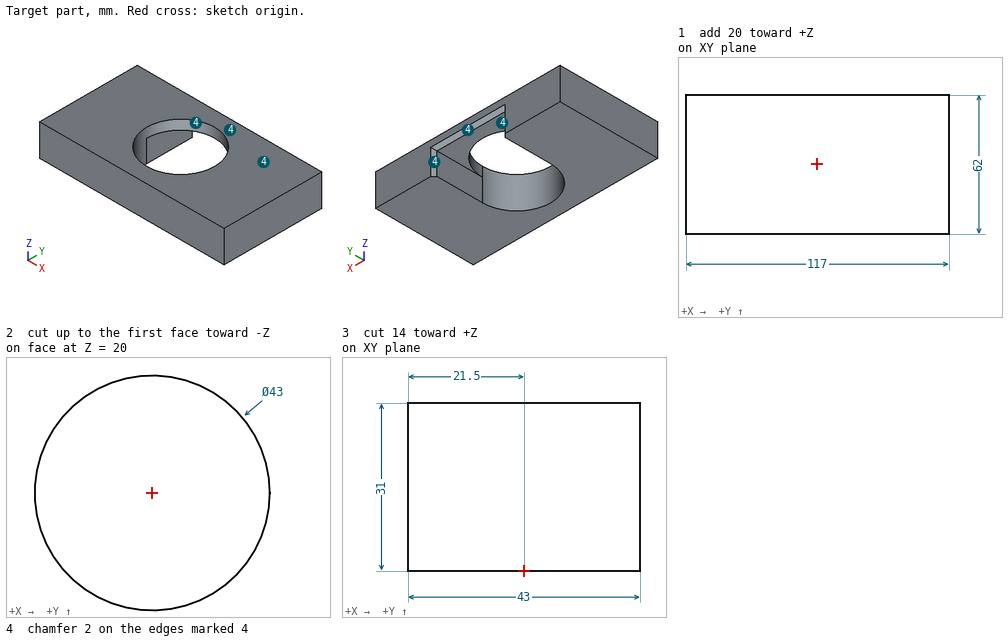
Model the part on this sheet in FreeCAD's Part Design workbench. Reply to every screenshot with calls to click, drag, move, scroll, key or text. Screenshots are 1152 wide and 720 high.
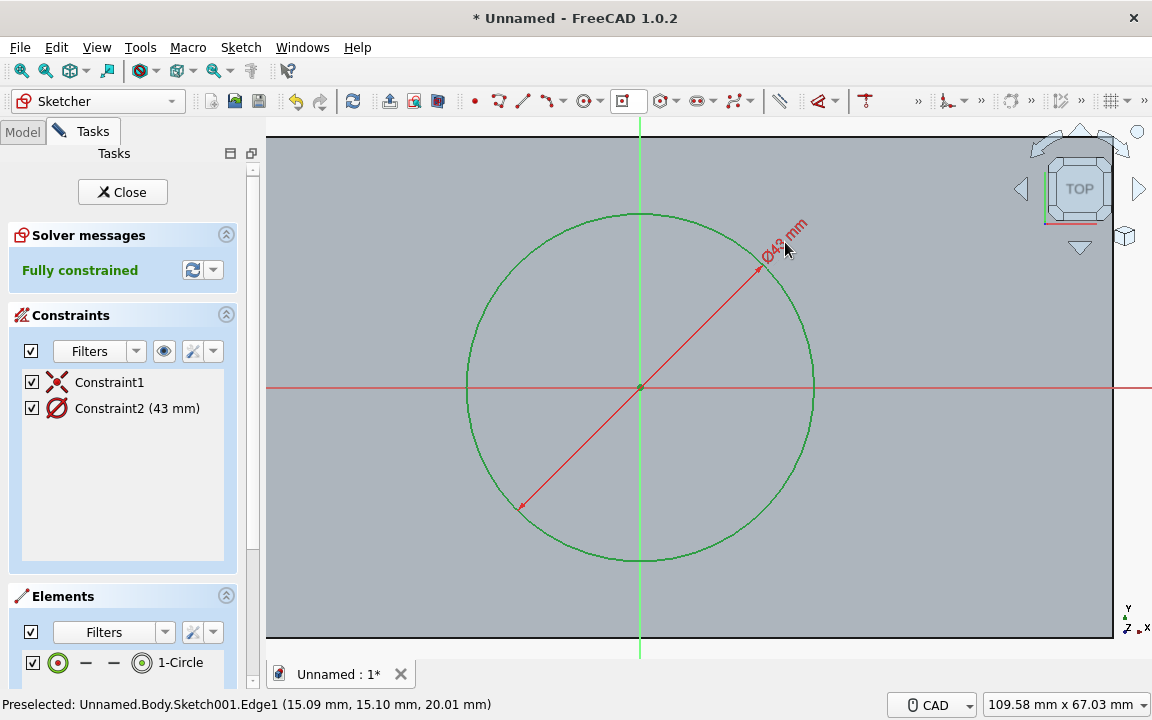
click(123, 192)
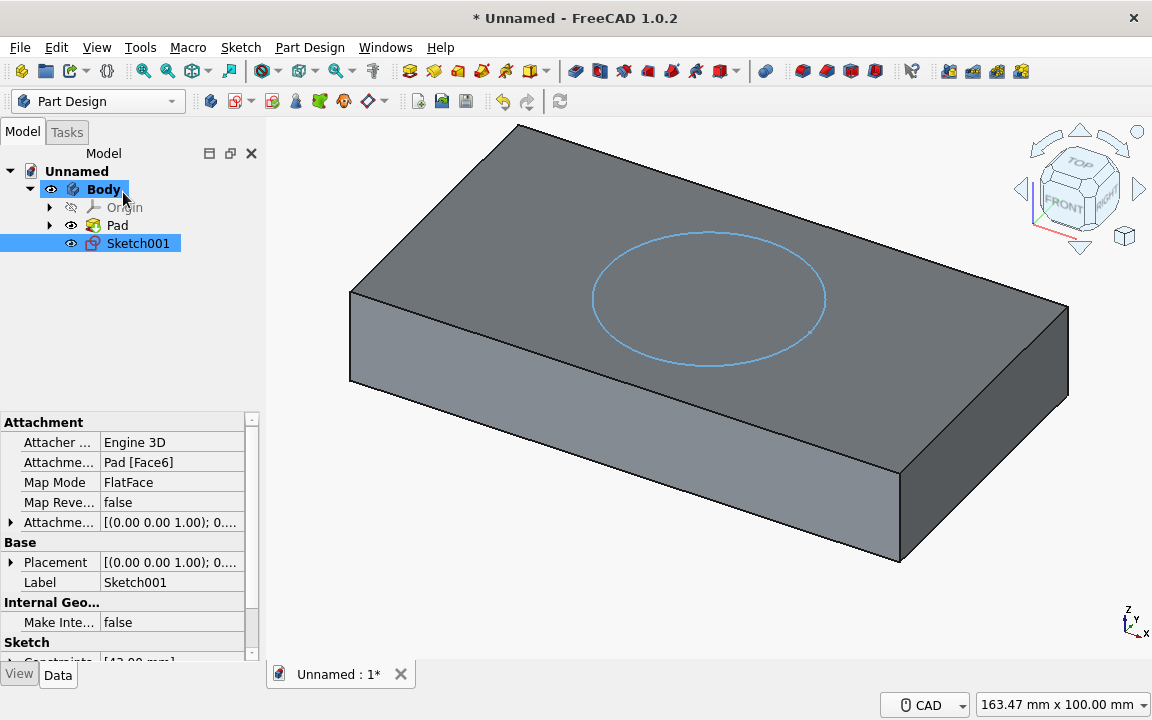
click(576, 72)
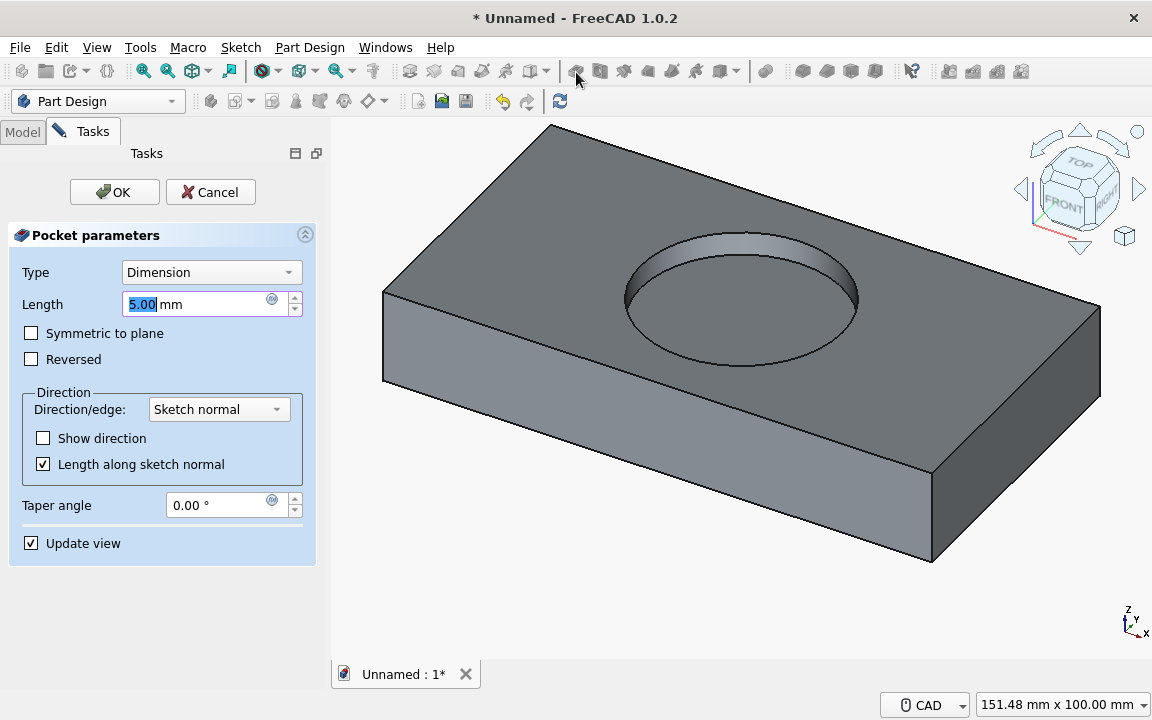
click(212, 272)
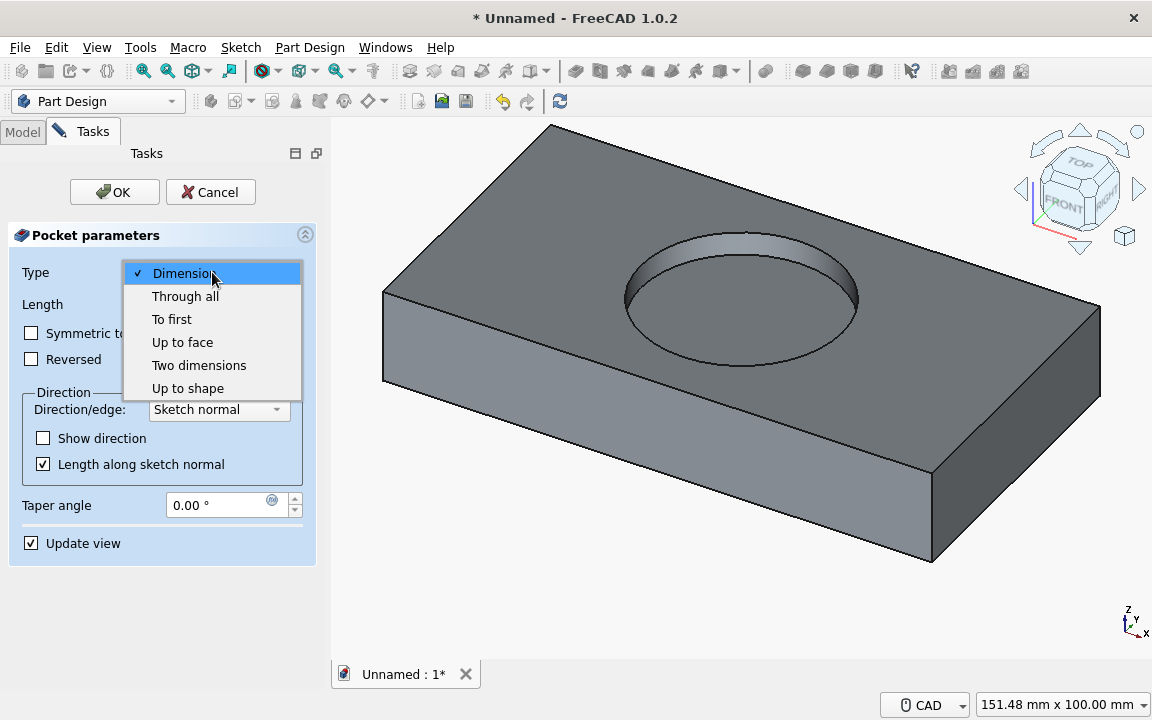
click(212, 320)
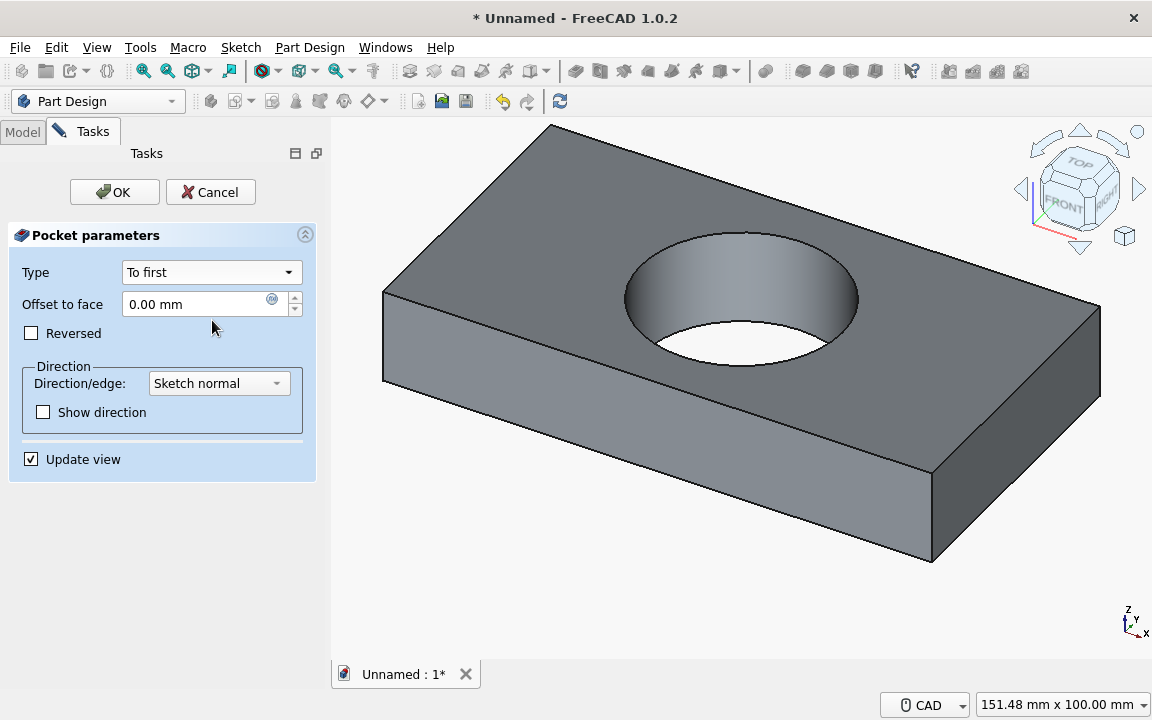
click(115, 192)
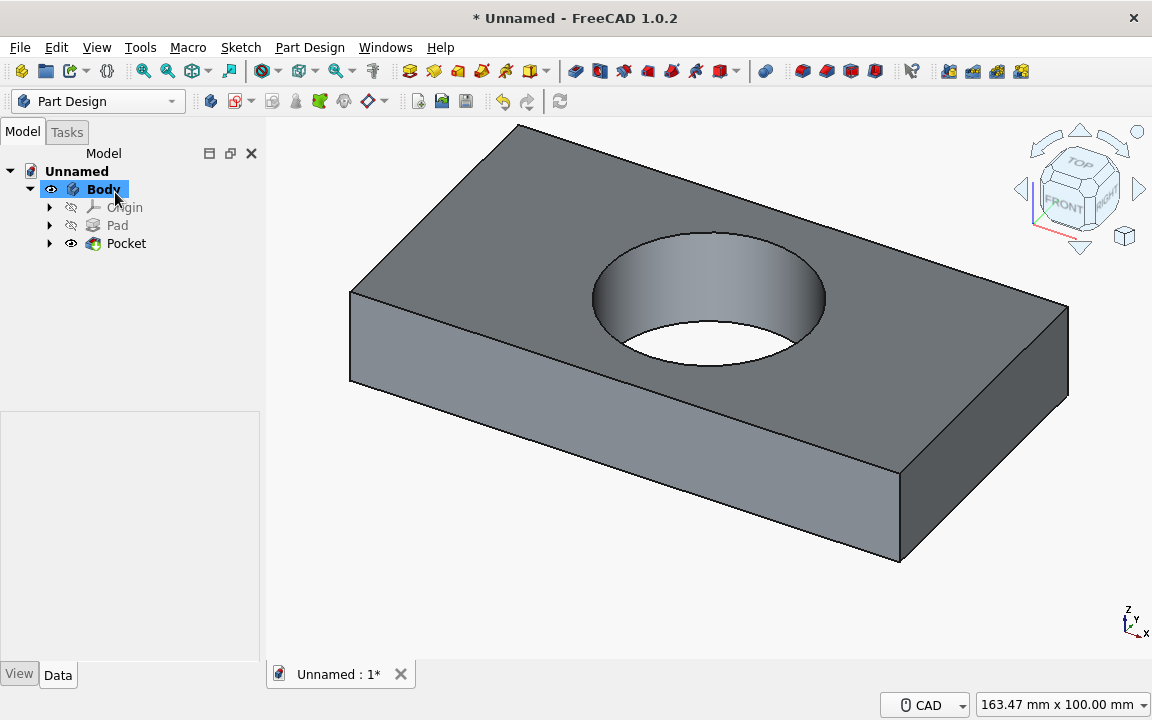
click(236, 102)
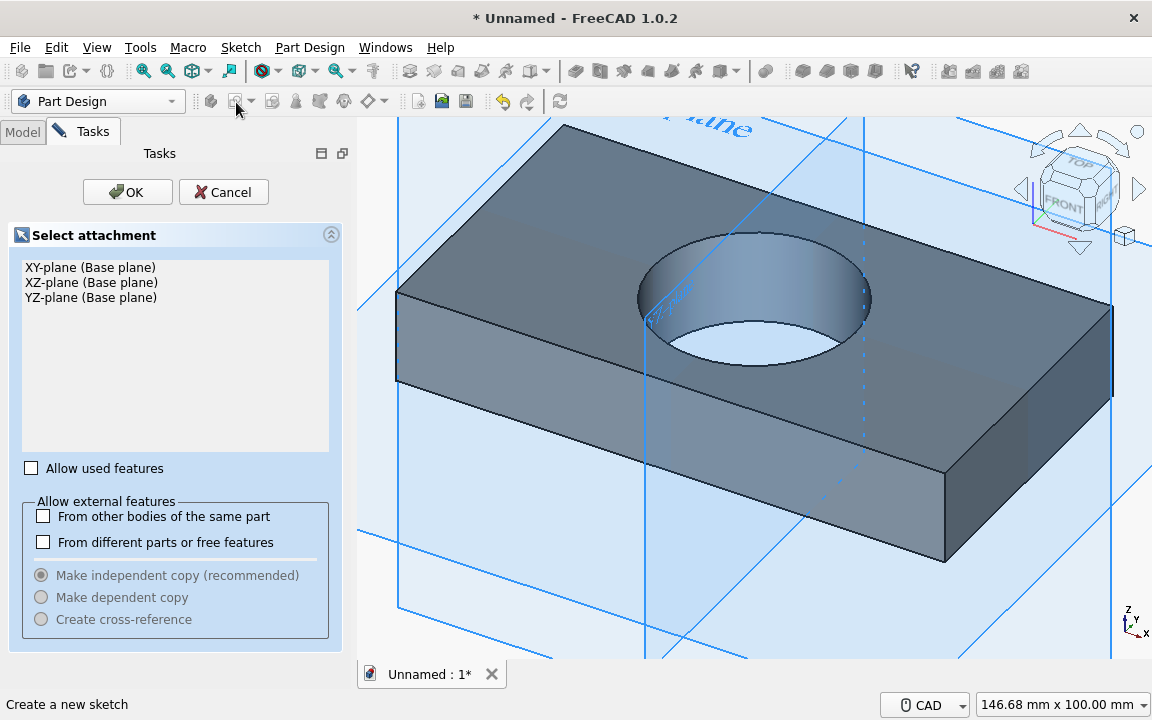
click(82, 268)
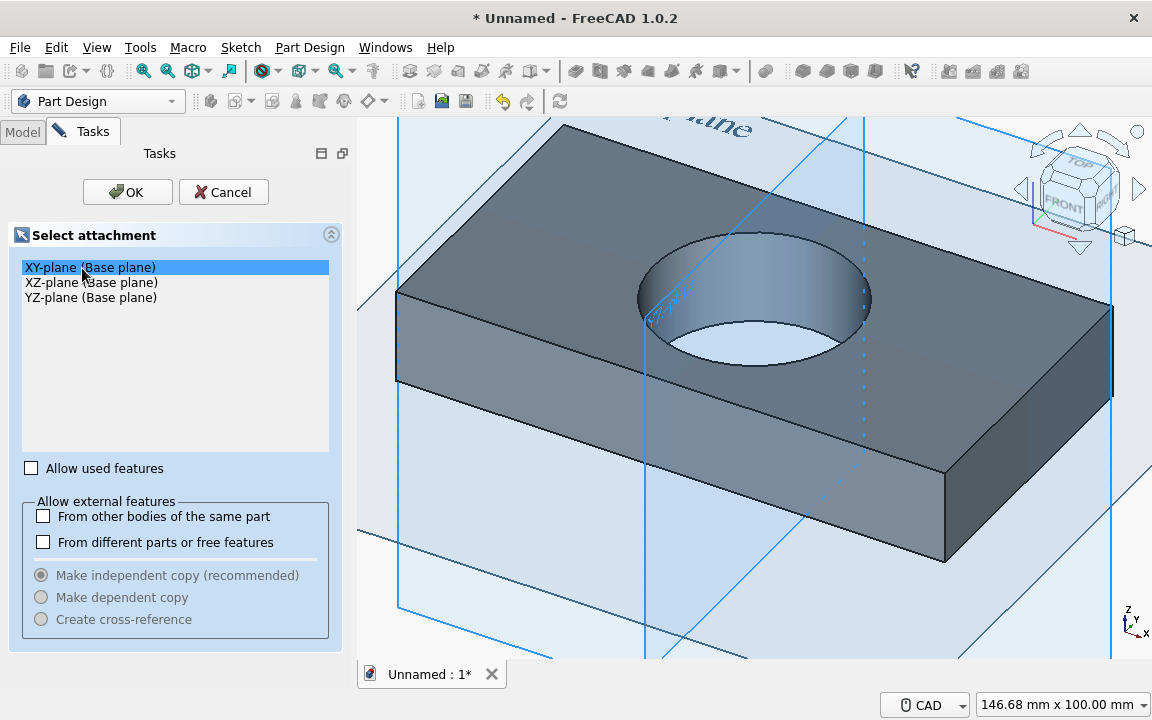
click(128, 192)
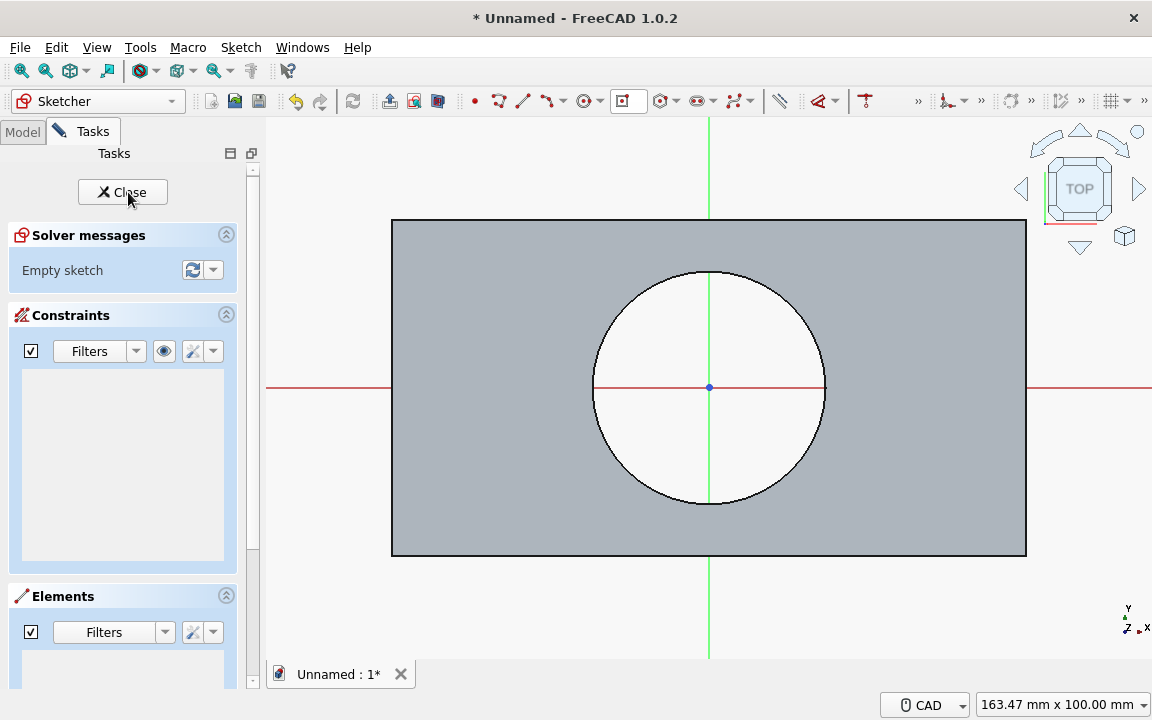
key(q)
key(s)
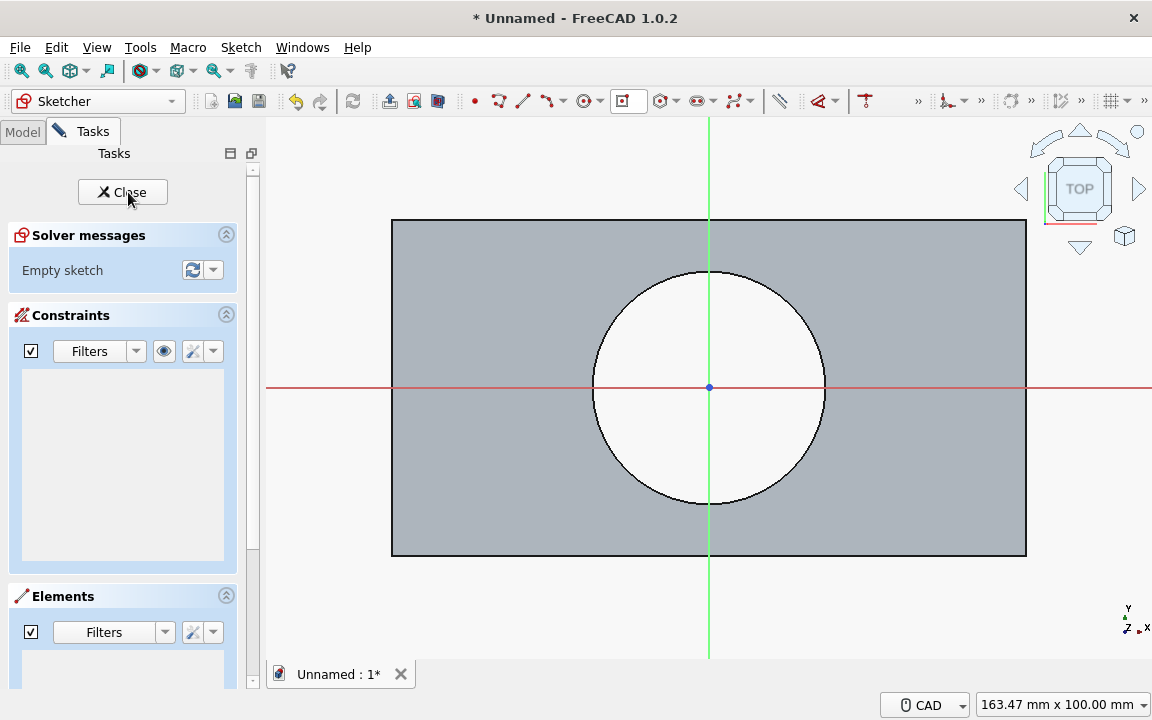
scroll(765, 235, up, 4)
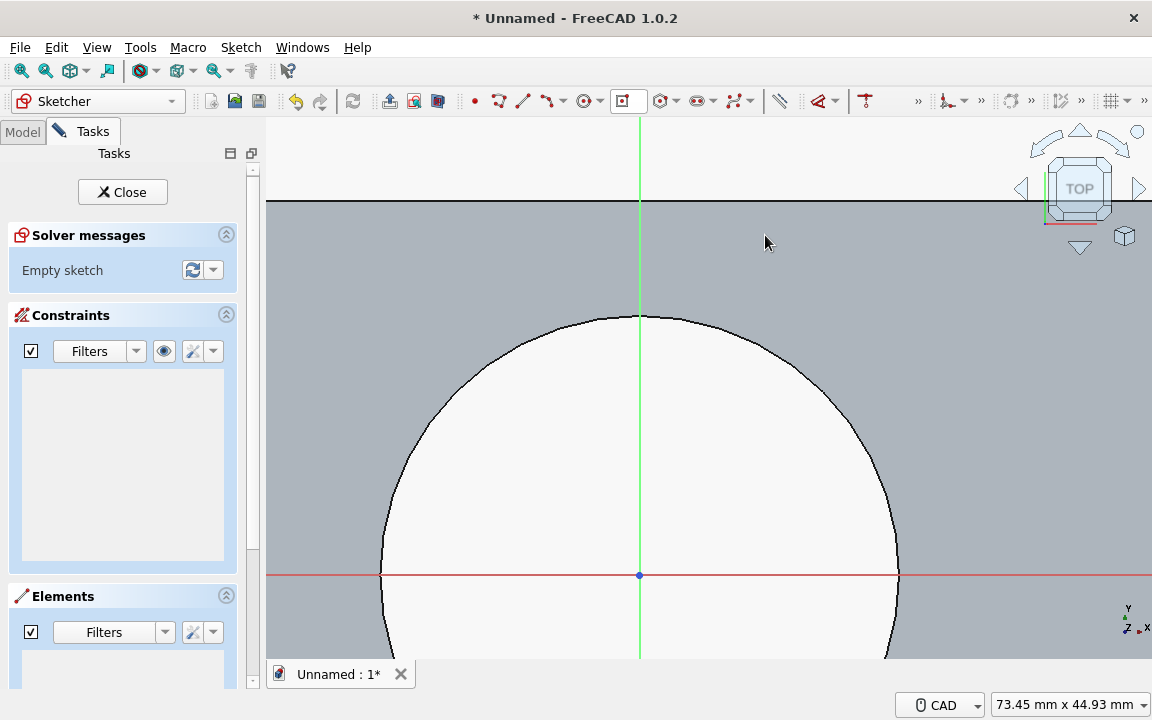
key(g)
key(r)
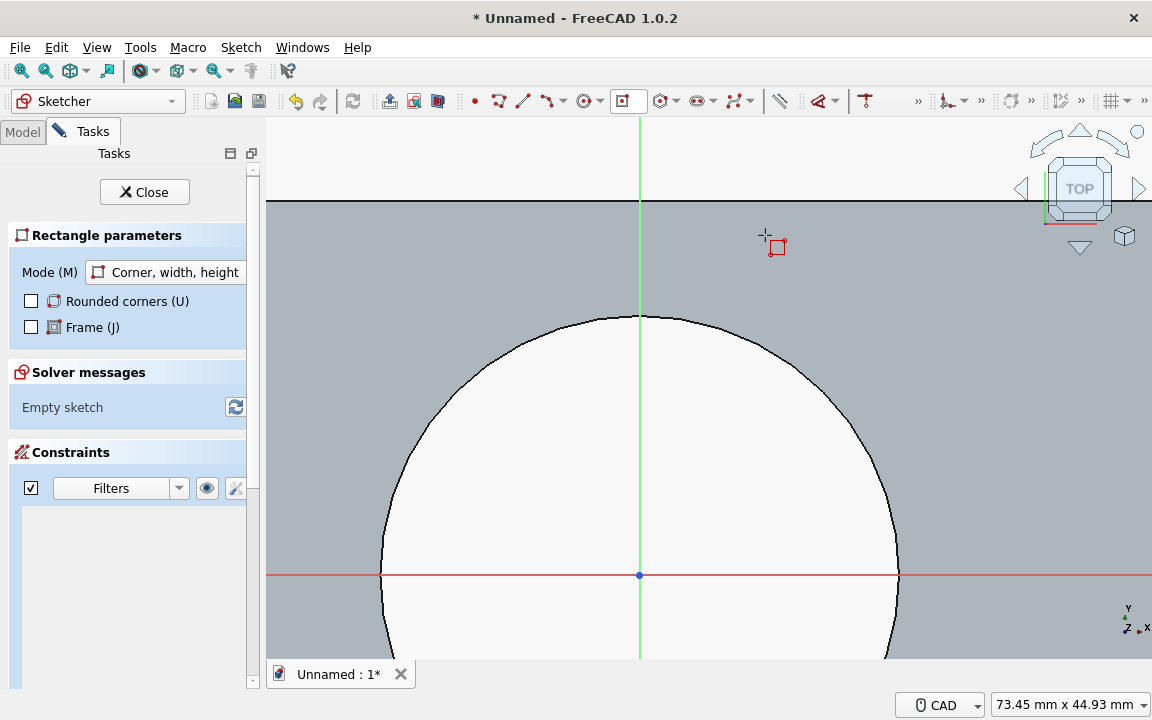
click(380, 201)
click(899, 575)
key(Escape)